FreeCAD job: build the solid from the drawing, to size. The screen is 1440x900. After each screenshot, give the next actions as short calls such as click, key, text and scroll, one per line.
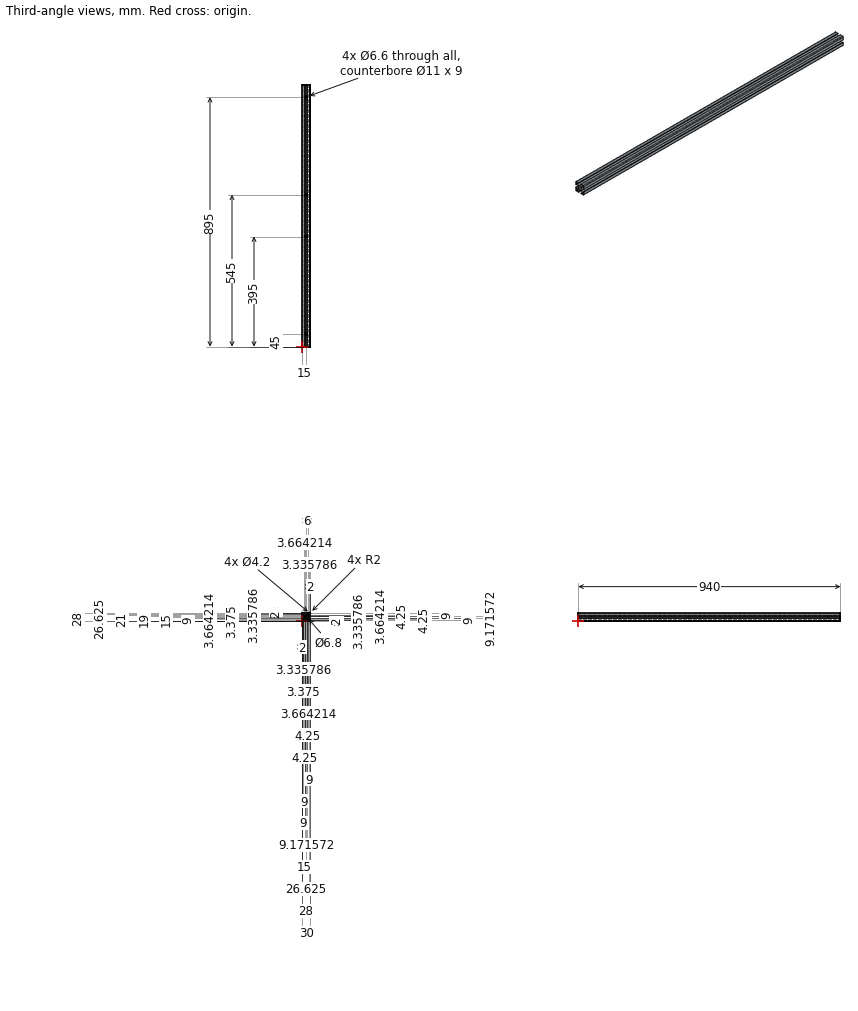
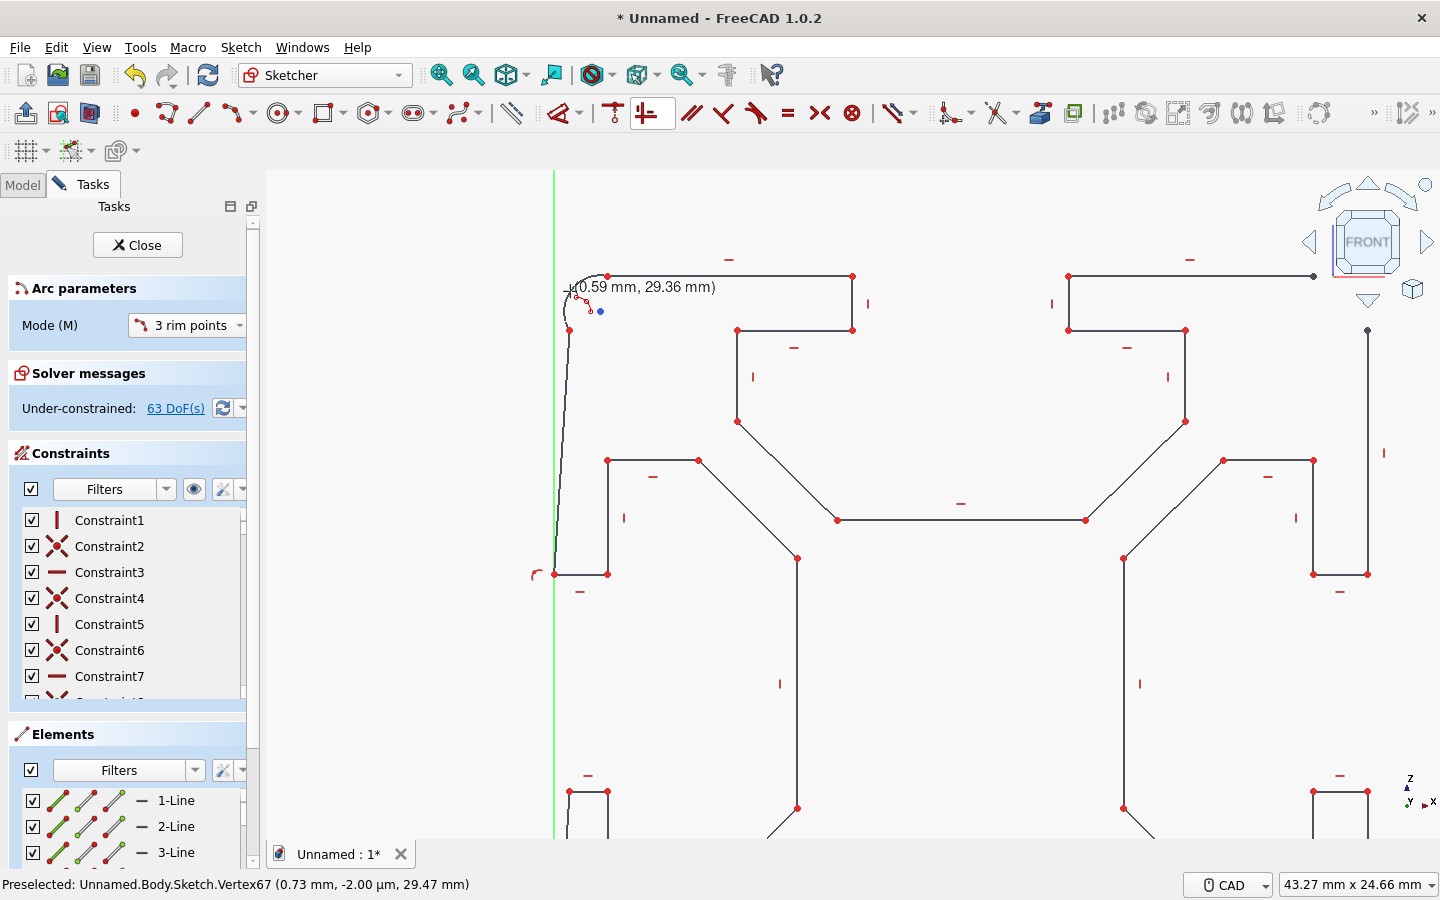
scroll(570, 289, down, 3)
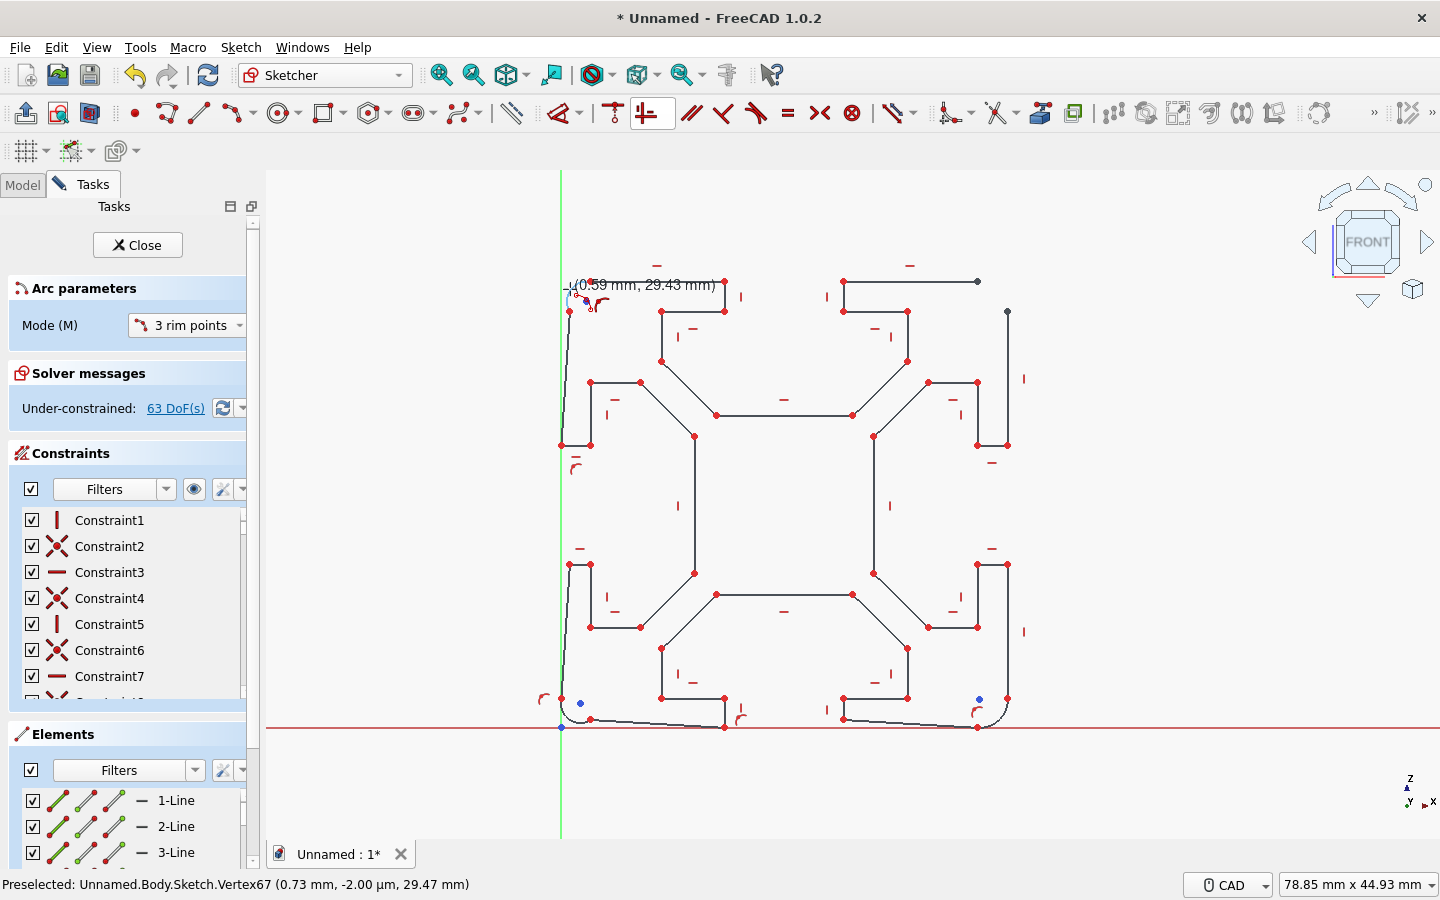
click(978, 282)
click(1008, 312)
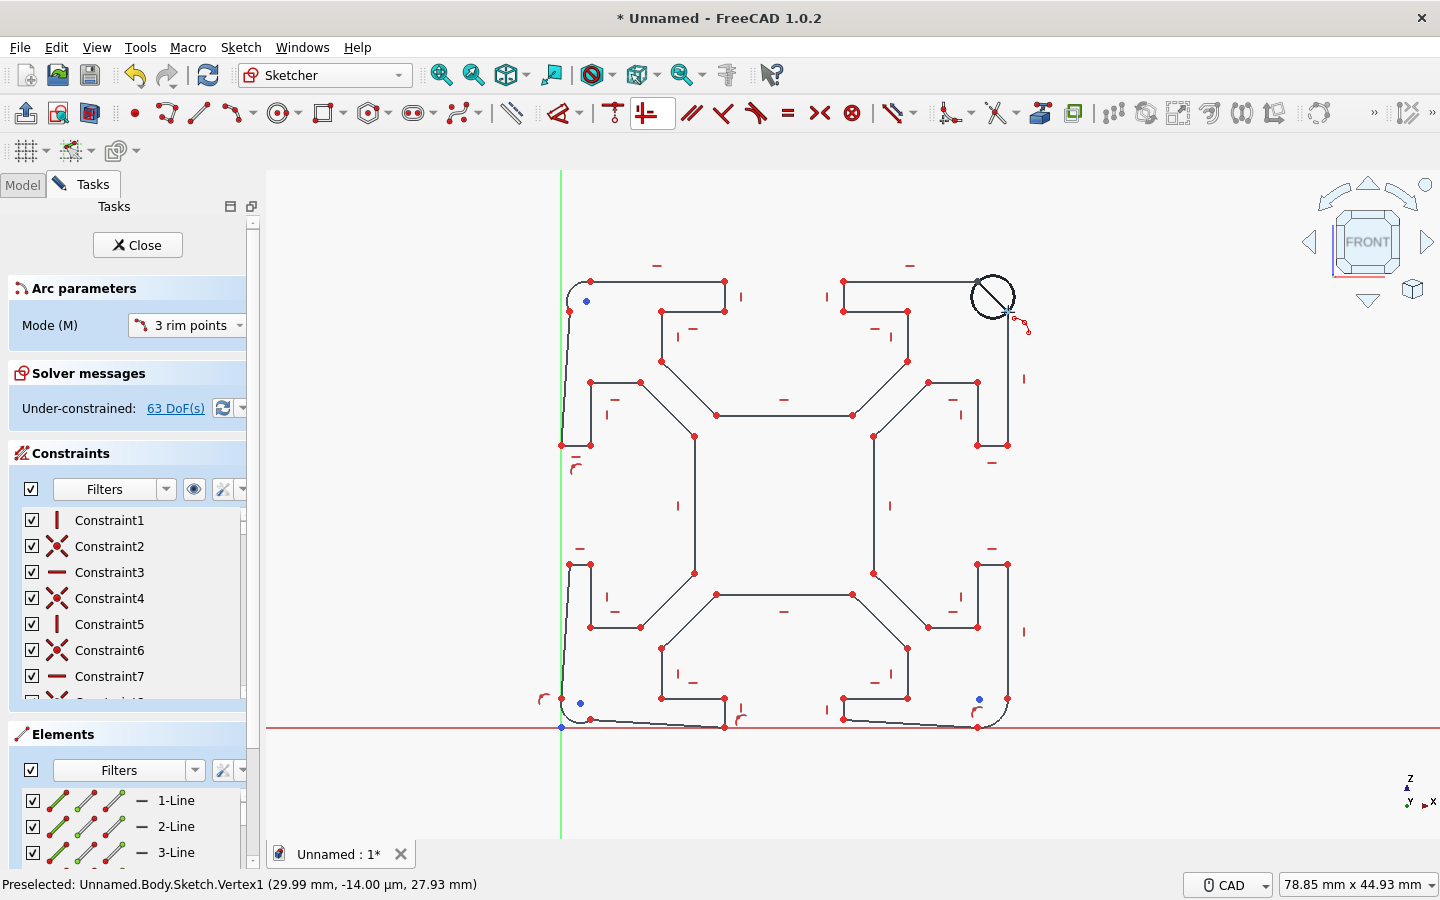
scroll(999, 290, up, 3)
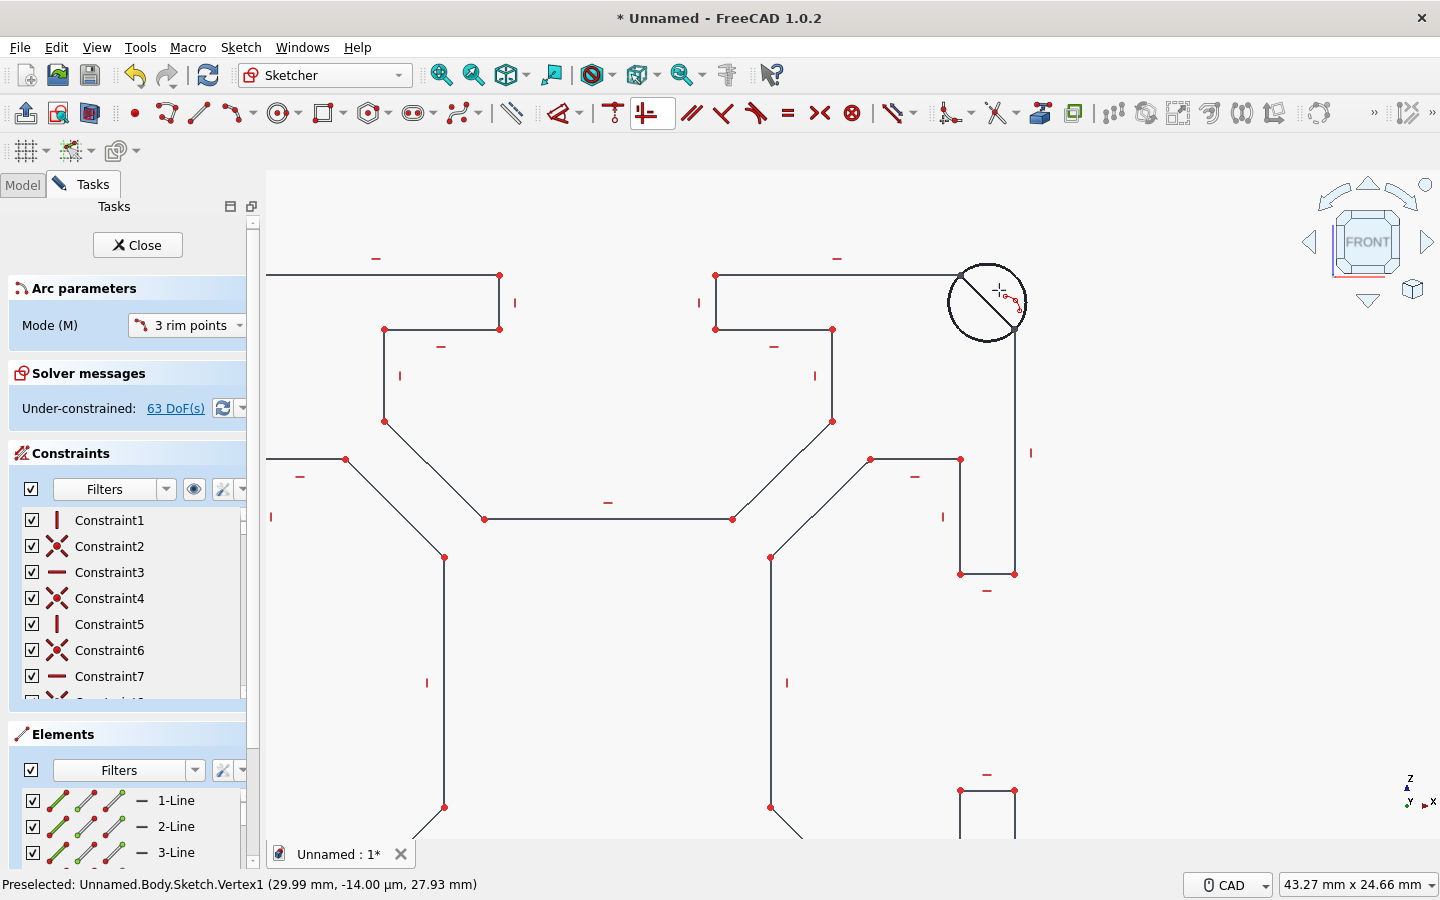
click(999, 290)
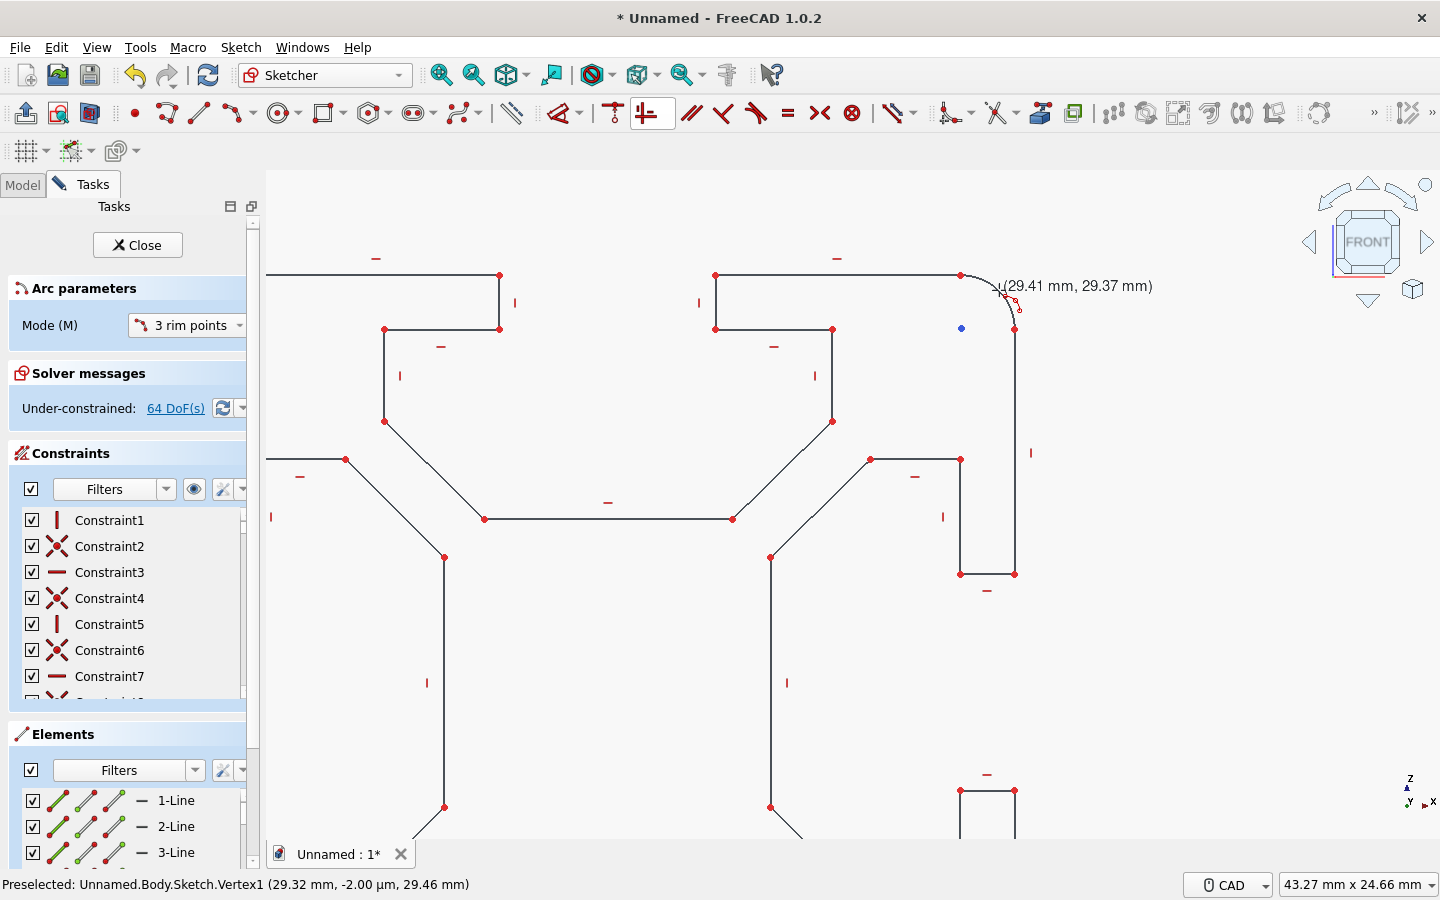
key(g)
key(c)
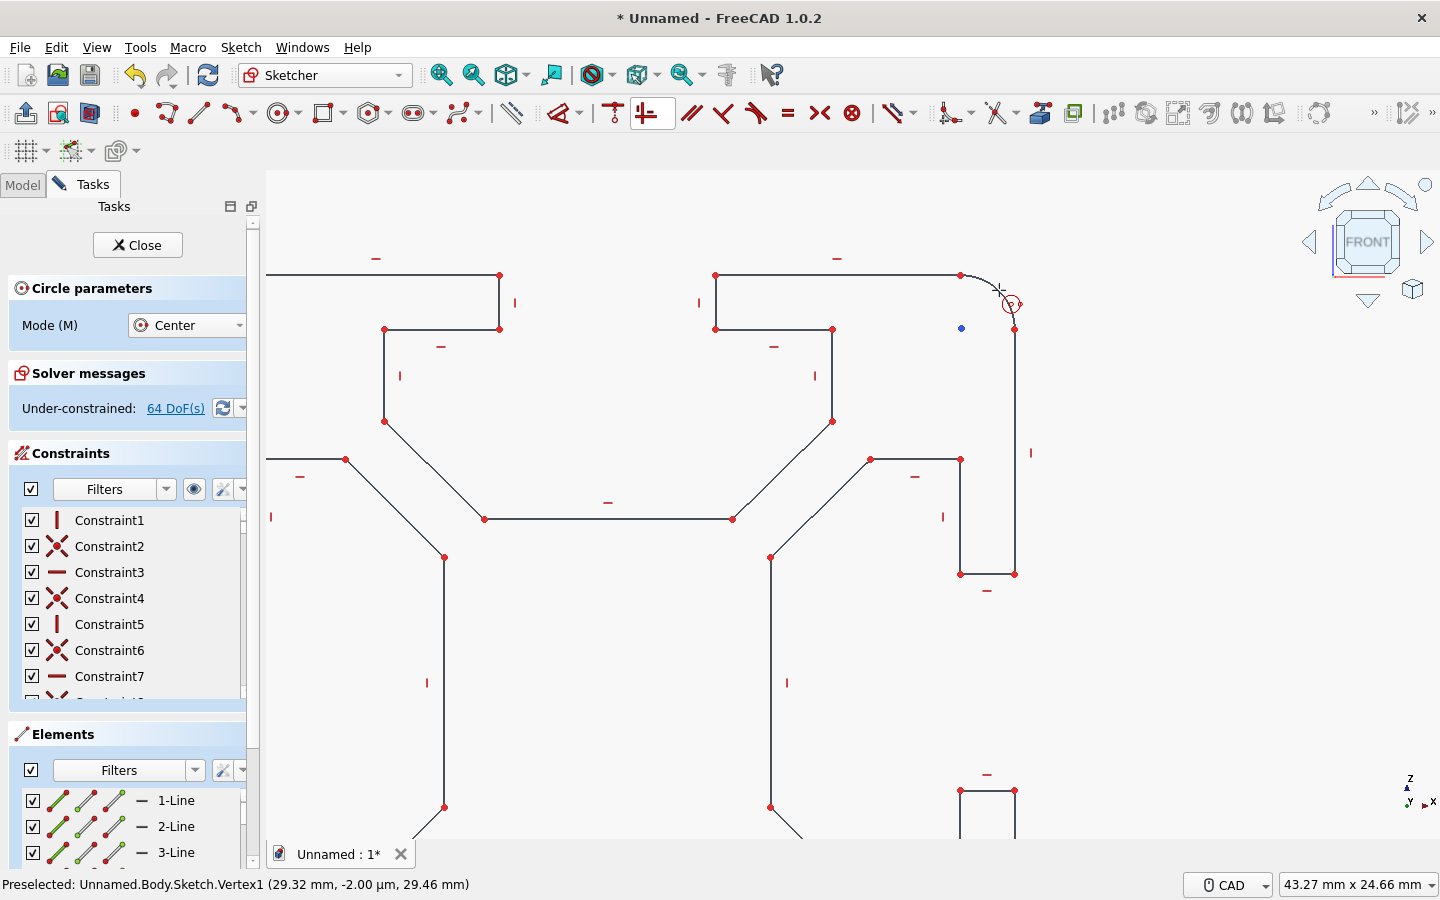
click(923, 365)
move(883, 325)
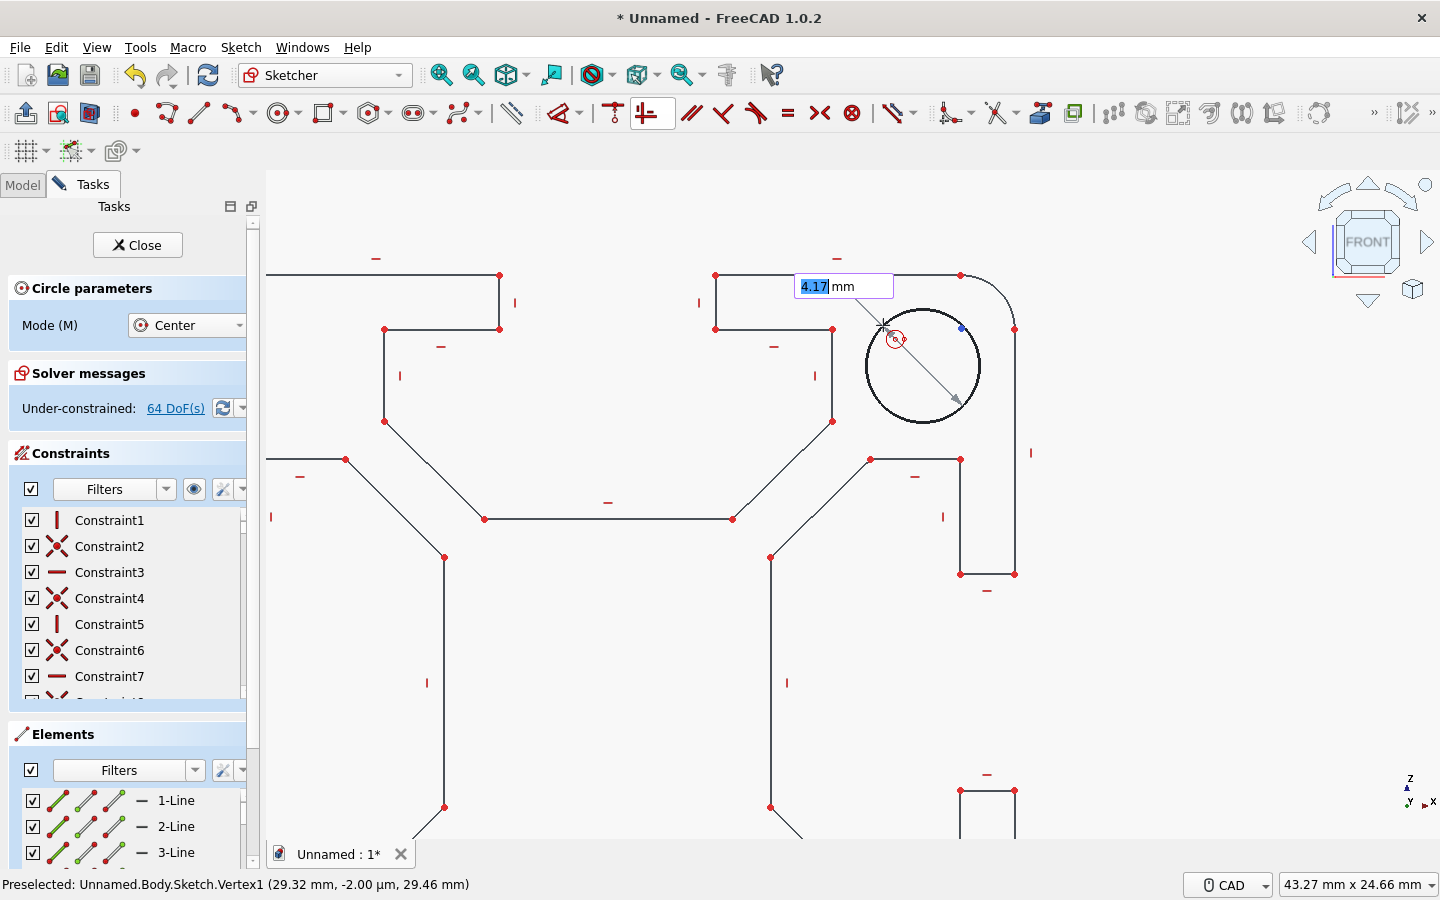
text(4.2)
key(Return)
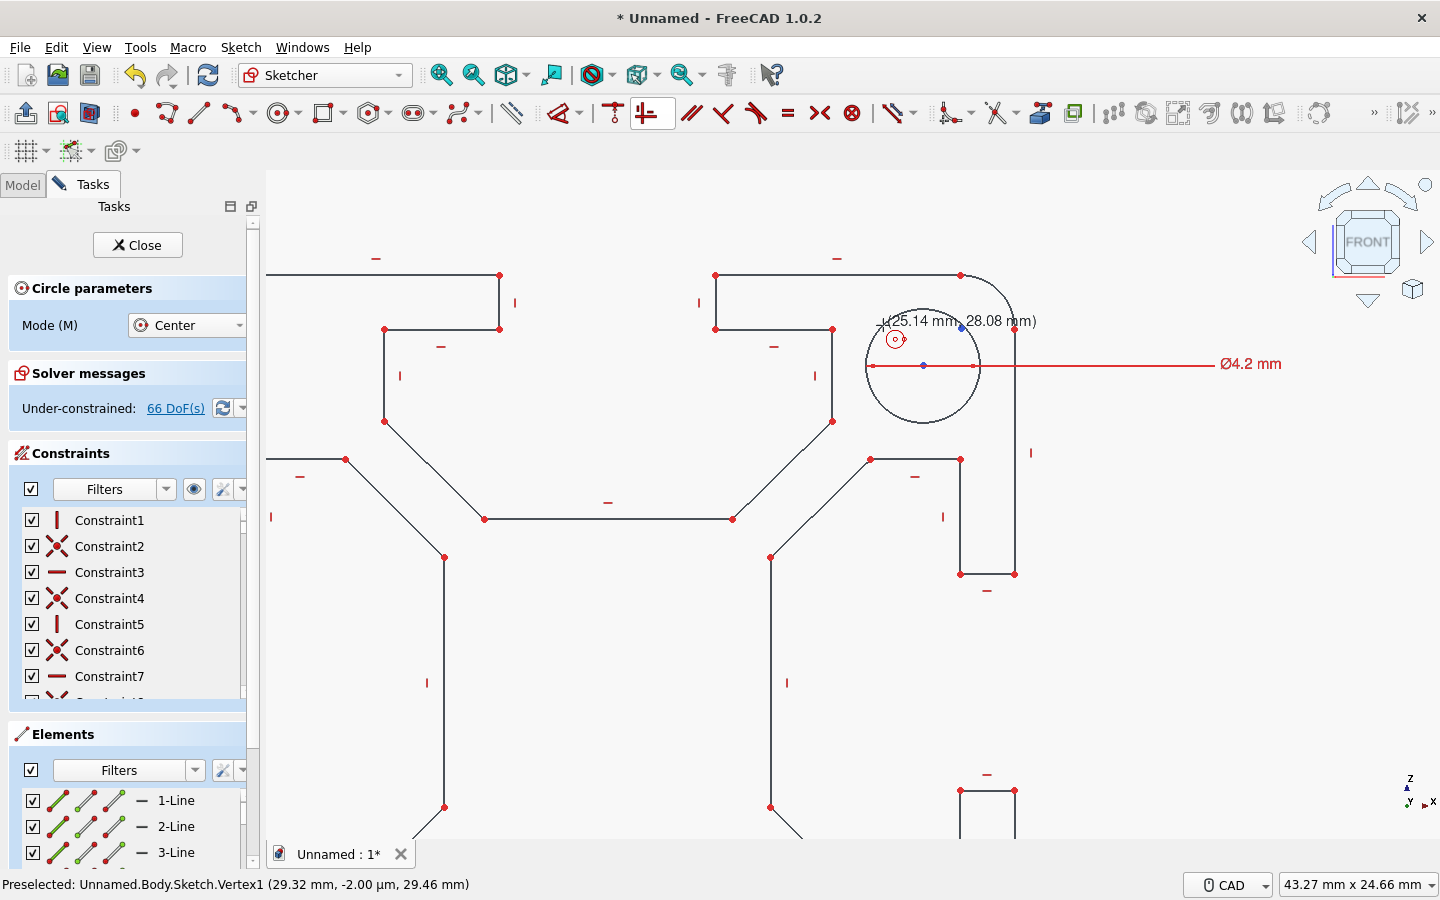
scroll(999, 290, down, 3)